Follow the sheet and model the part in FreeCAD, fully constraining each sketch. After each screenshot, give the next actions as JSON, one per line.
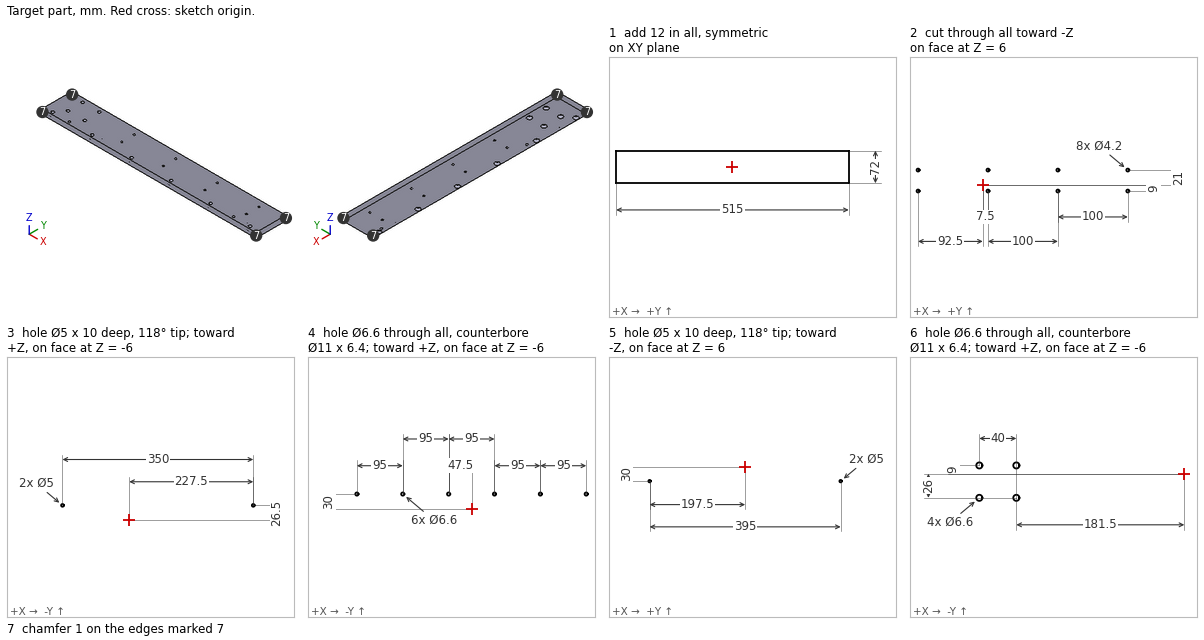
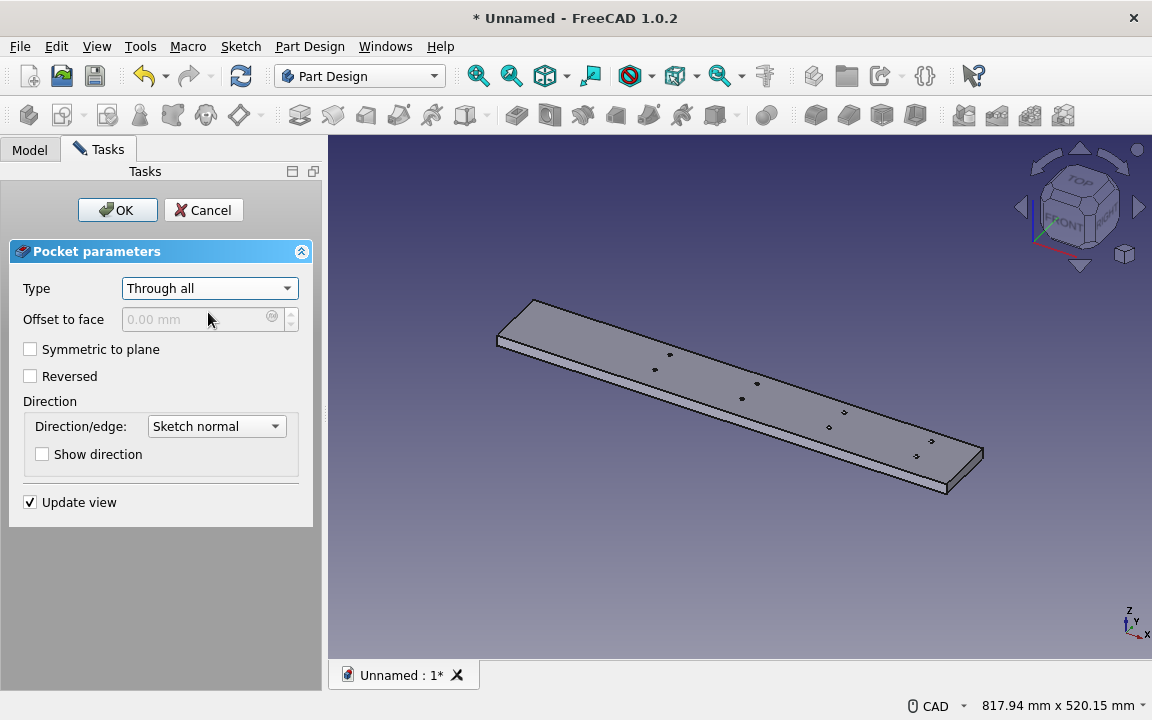
{"action": "left_click", "coordinate": [118, 210]}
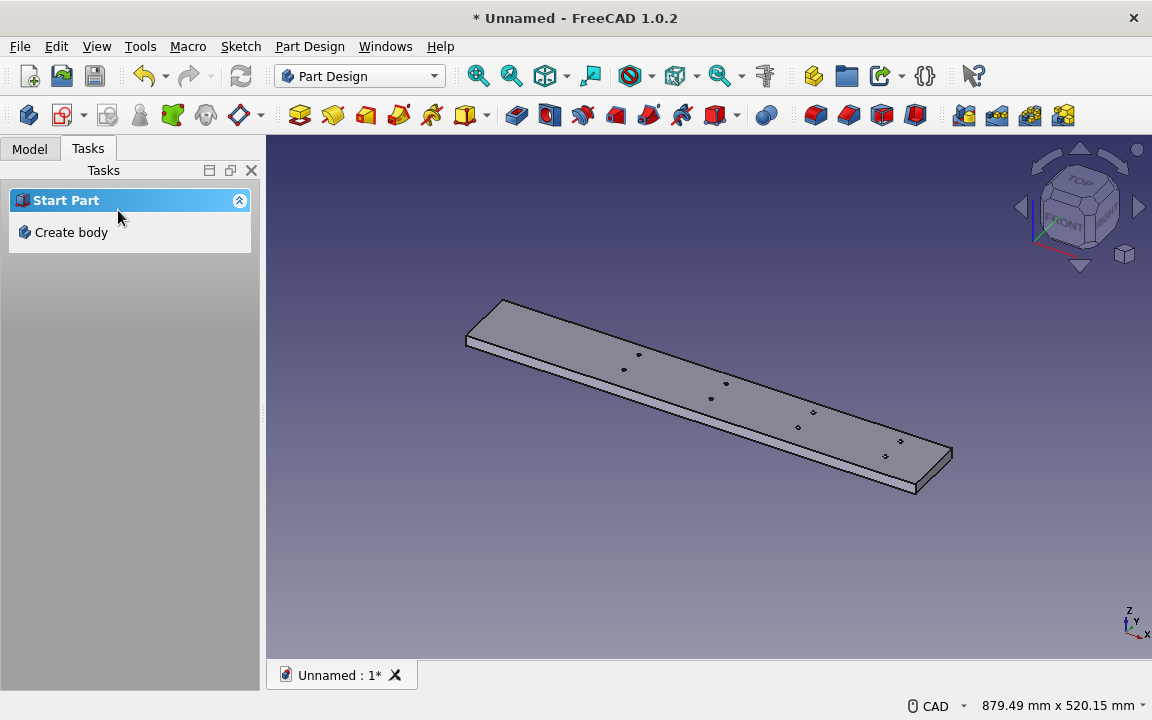
{"action": "key", "text": "5"}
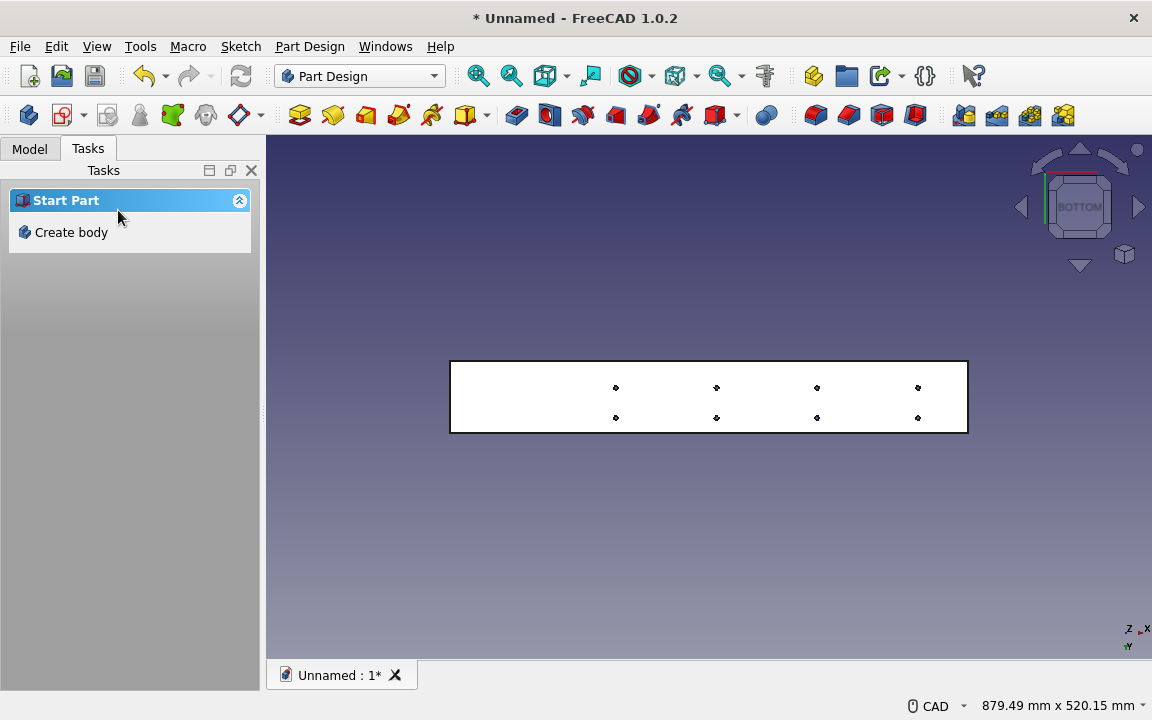
{"action": "left_click", "coordinate": [857, 396]}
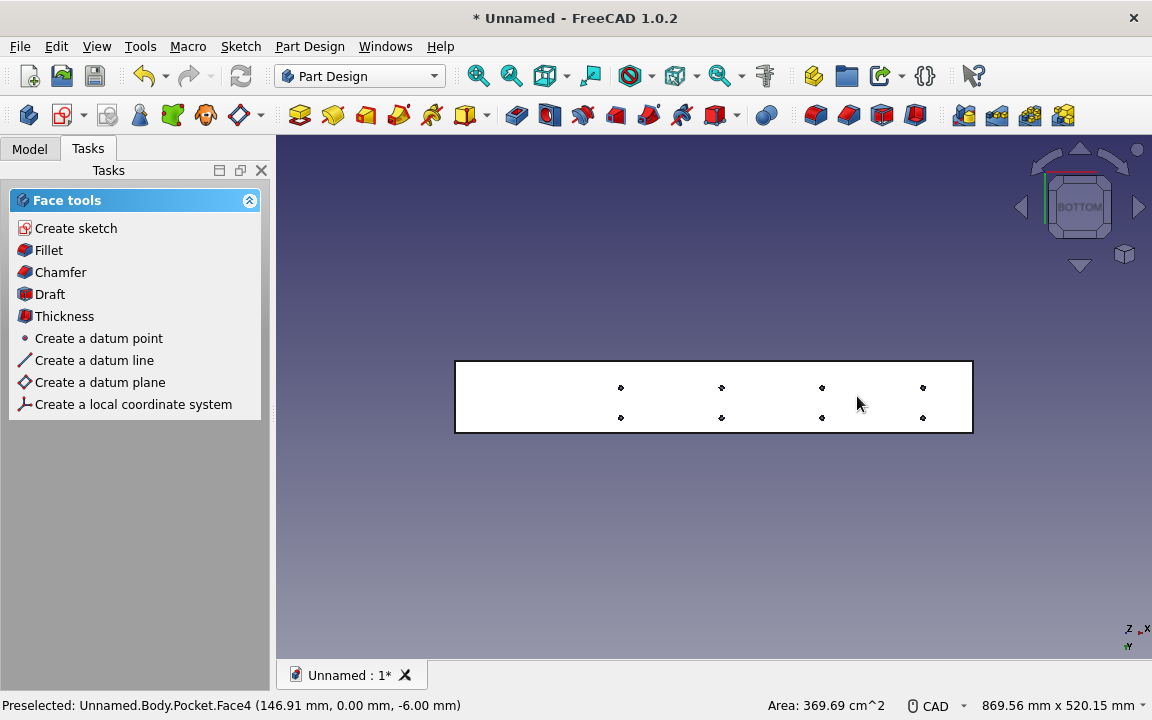
{"action": "left_click", "coordinate": [62, 116]}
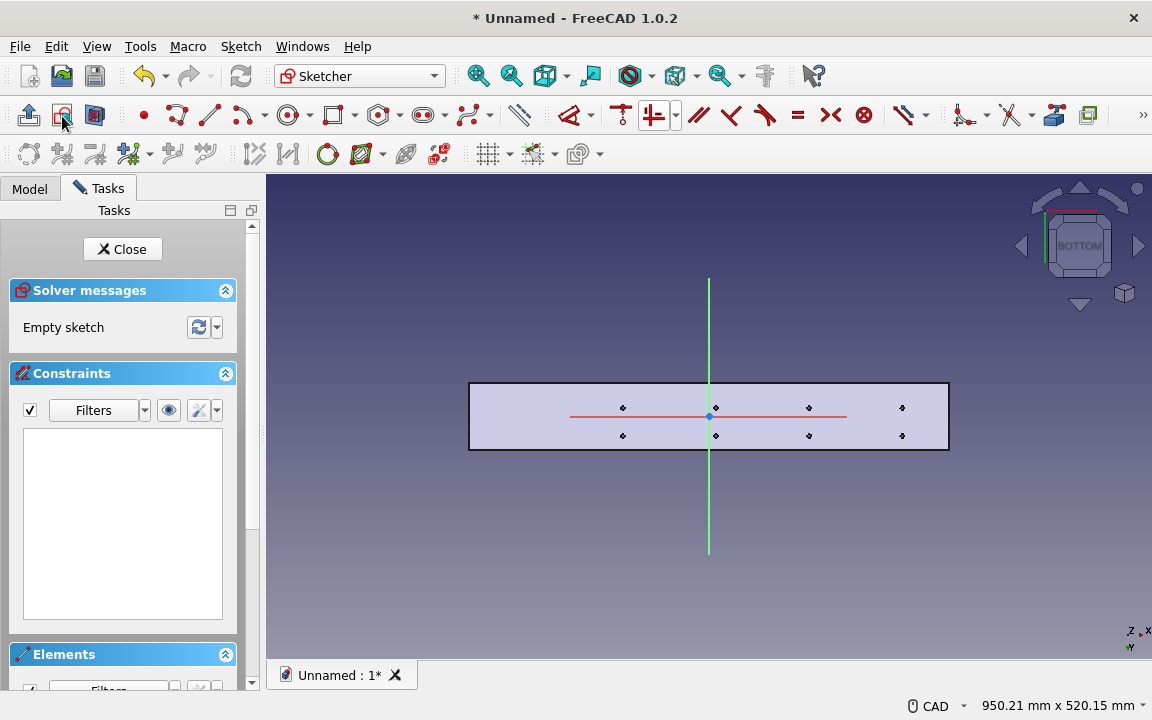
{"action": "scroll", "coordinate": [987, 375], "scroll_direction": "up", "scroll_amount": 2}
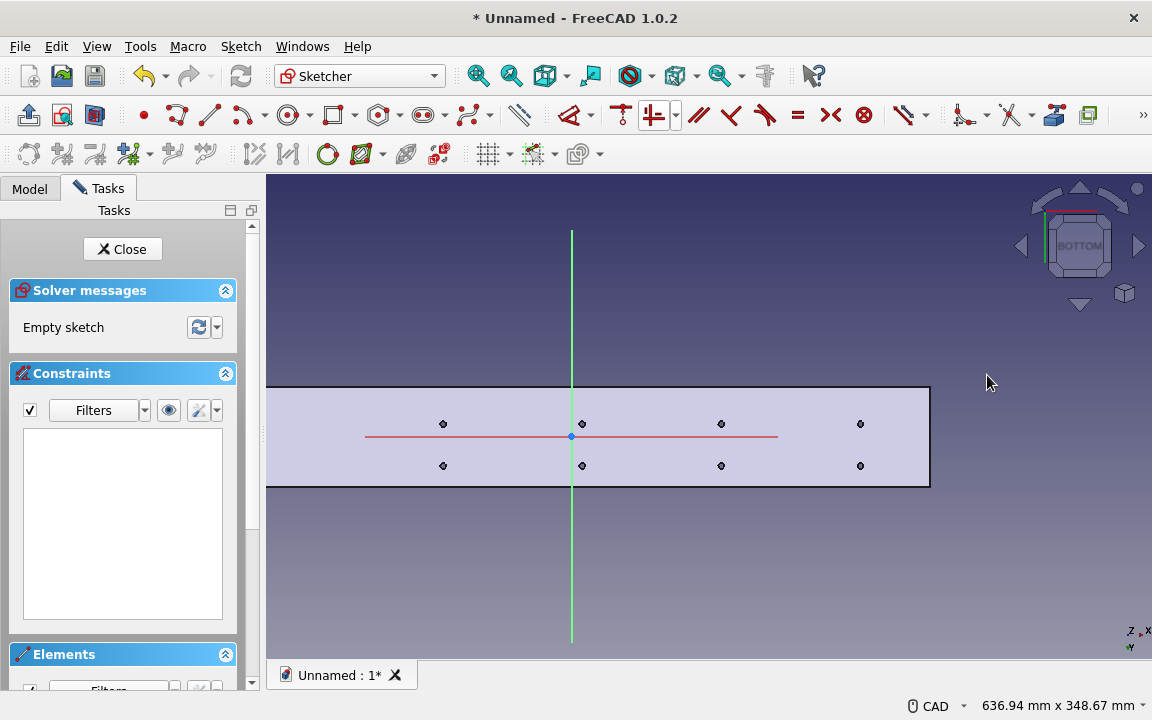
{"action": "left_click", "coordinate": [288, 116]}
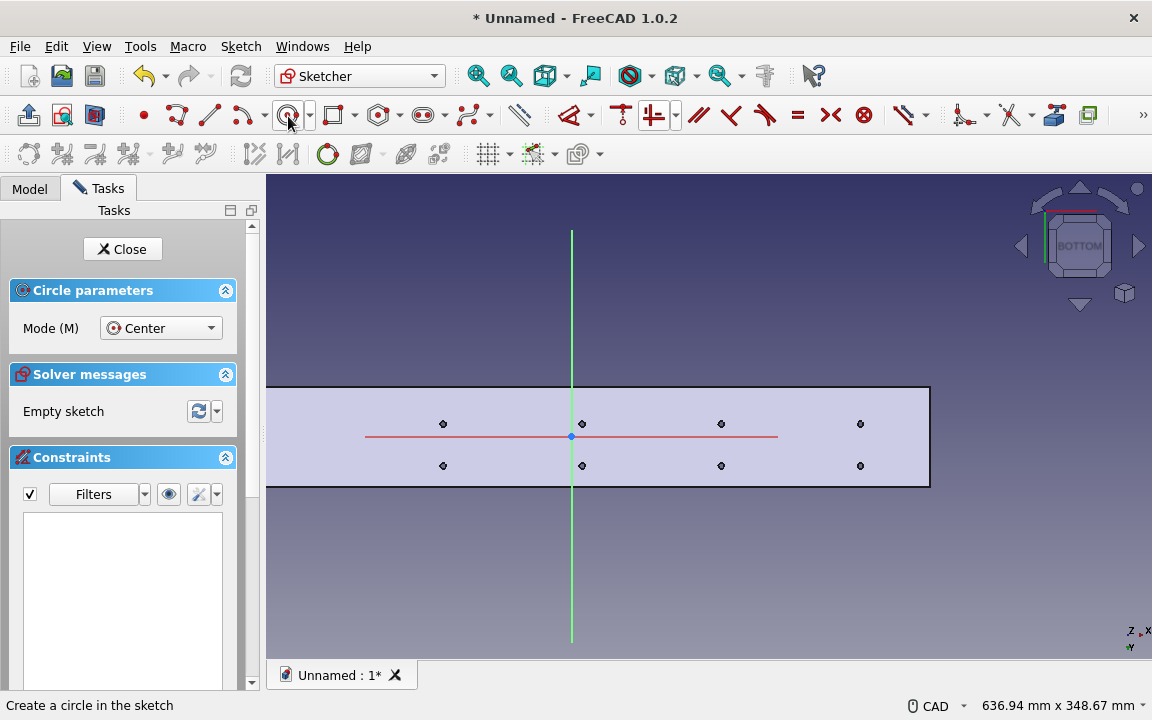
{"action": "scroll", "coordinate": [888, 400], "scroll_direction": "up", "scroll_amount": 10}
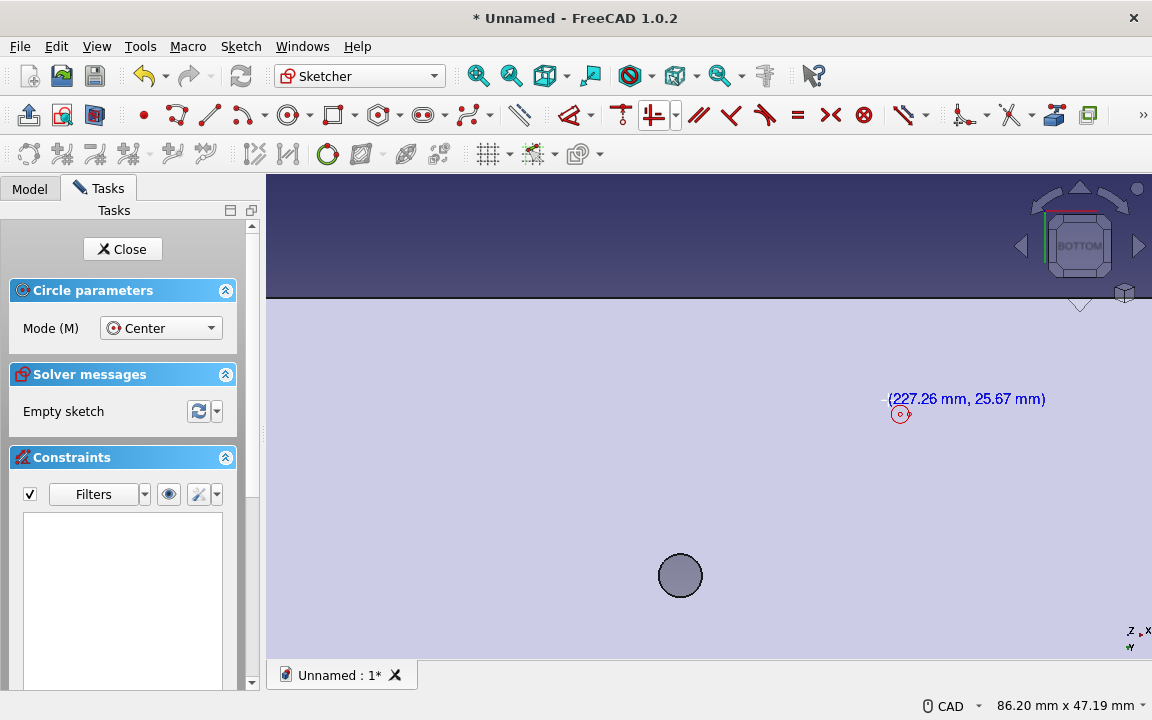
{"action": "scroll", "coordinate": [884, 400], "scroll_direction": "down", "scroll_amount": 10}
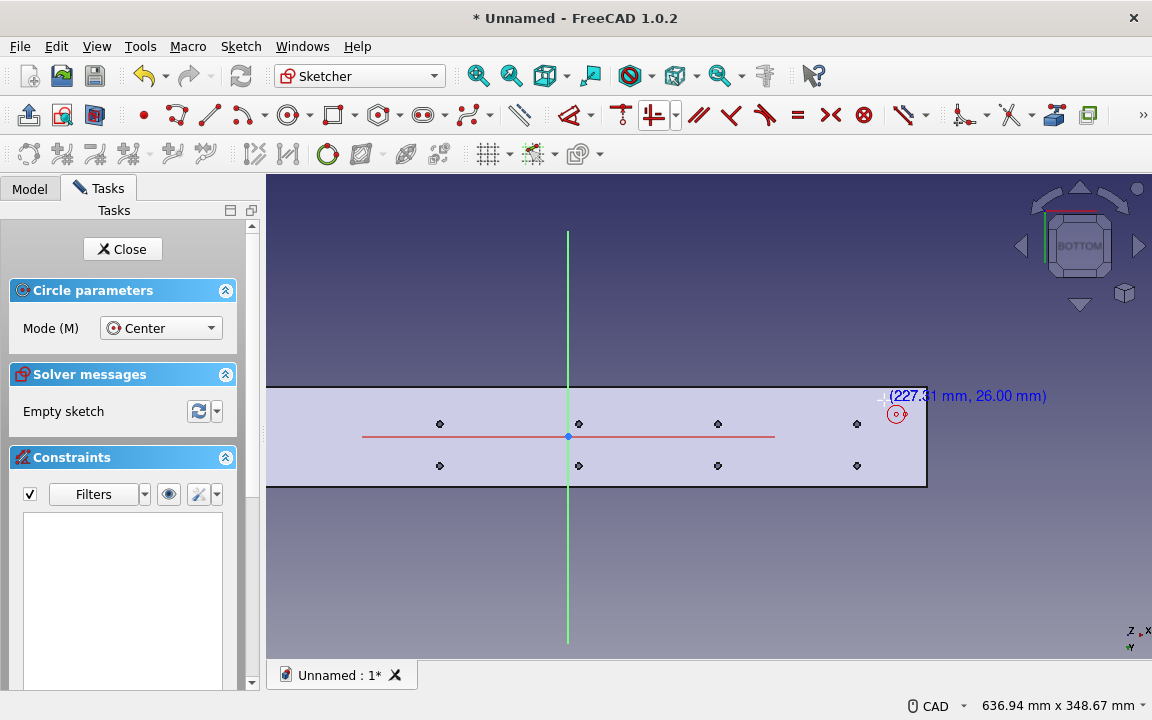
{"action": "left_click", "coordinate": [885, 400]}
{"action": "mouse_move", "coordinate": [887, 397]}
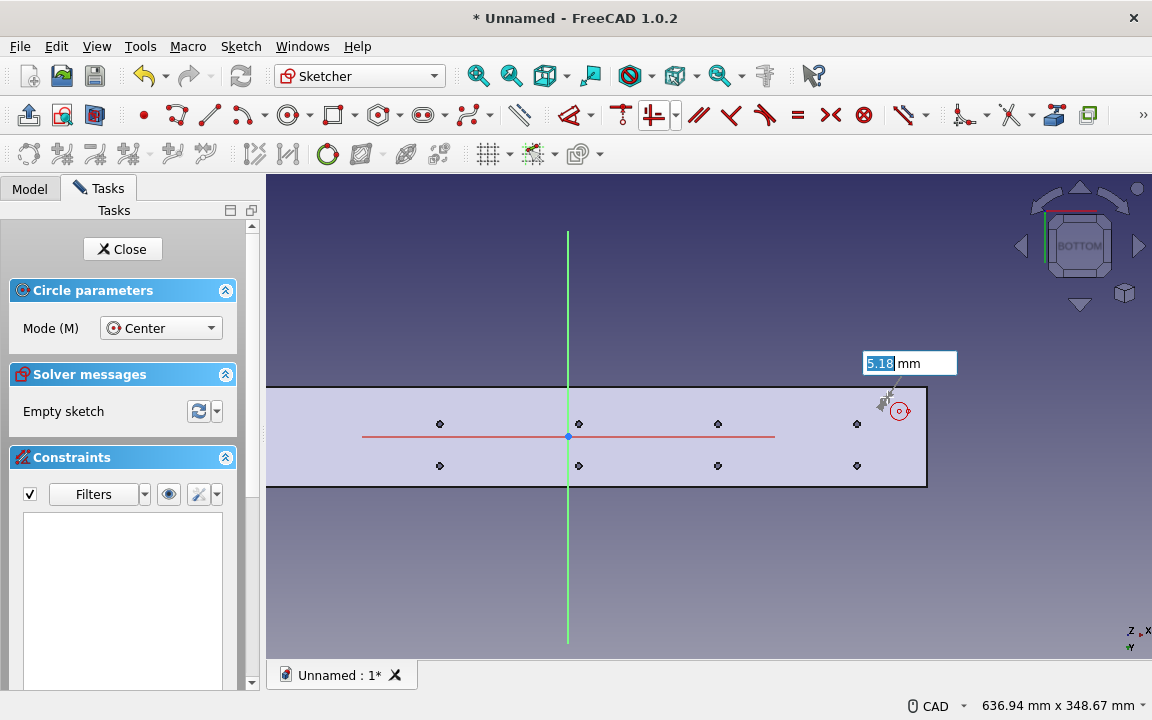
{"action": "type", "text": "5"}
{"action": "key", "text": "Return"}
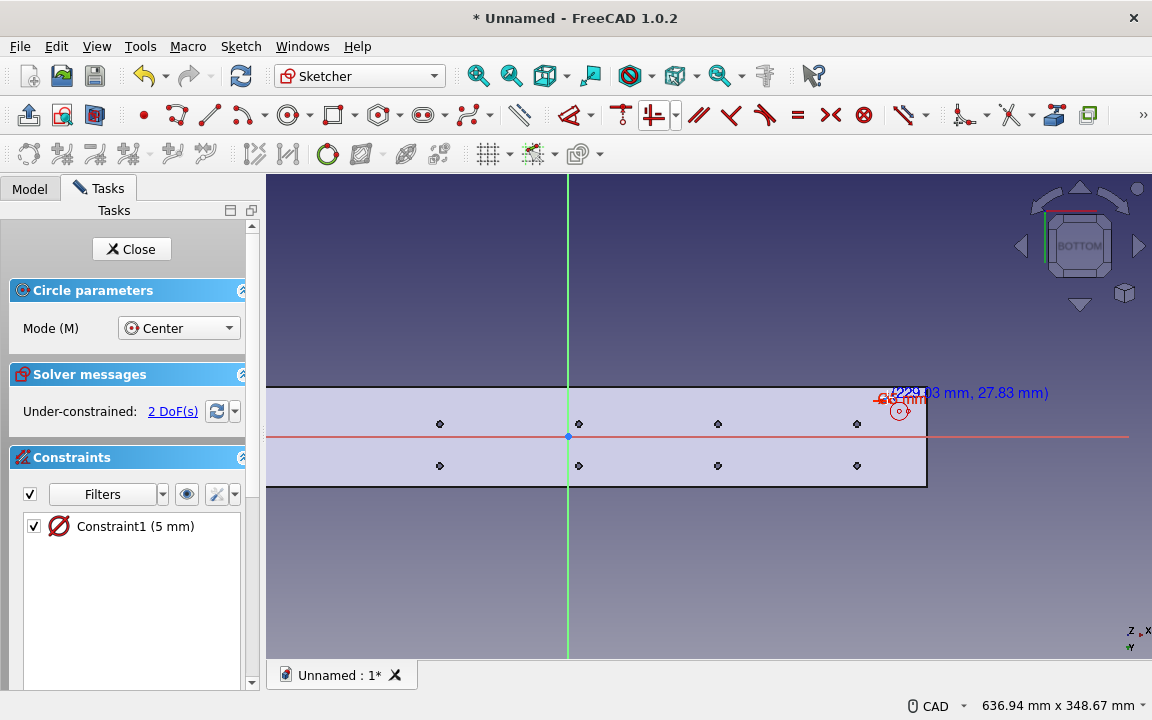
{"action": "scroll", "coordinate": [398, 400], "scroll_direction": "up", "scroll_amount": 10}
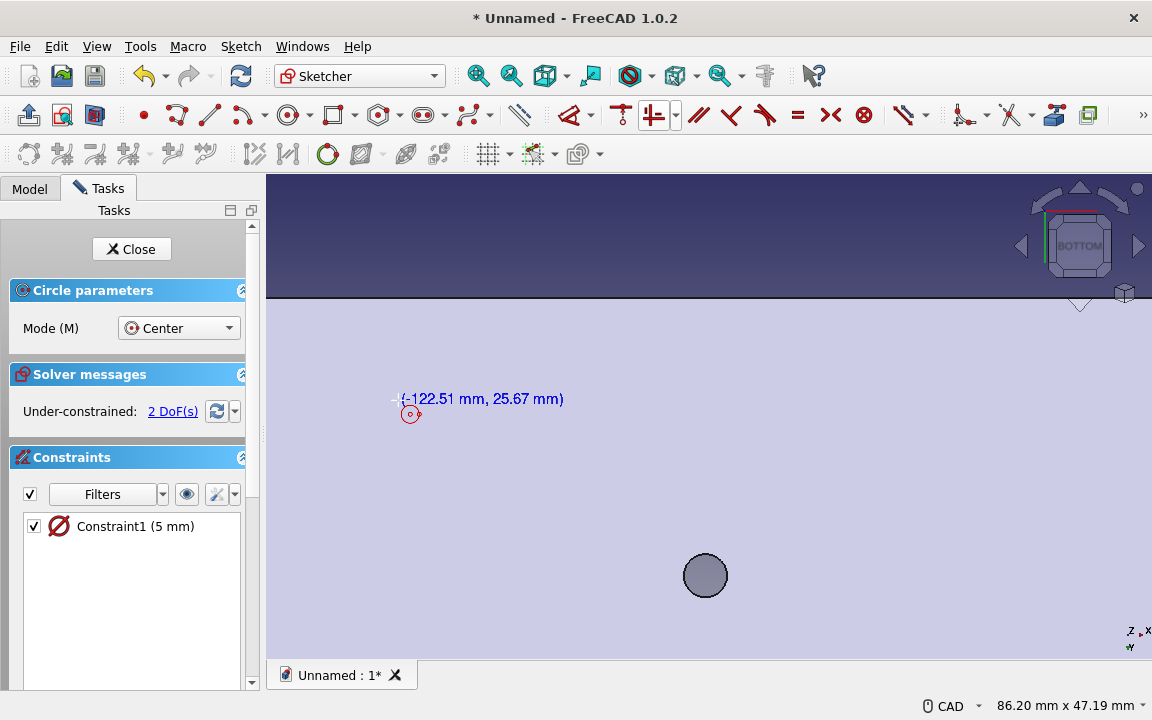
{"action": "scroll", "coordinate": [397, 400], "scroll_direction": "down", "scroll_amount": 10}